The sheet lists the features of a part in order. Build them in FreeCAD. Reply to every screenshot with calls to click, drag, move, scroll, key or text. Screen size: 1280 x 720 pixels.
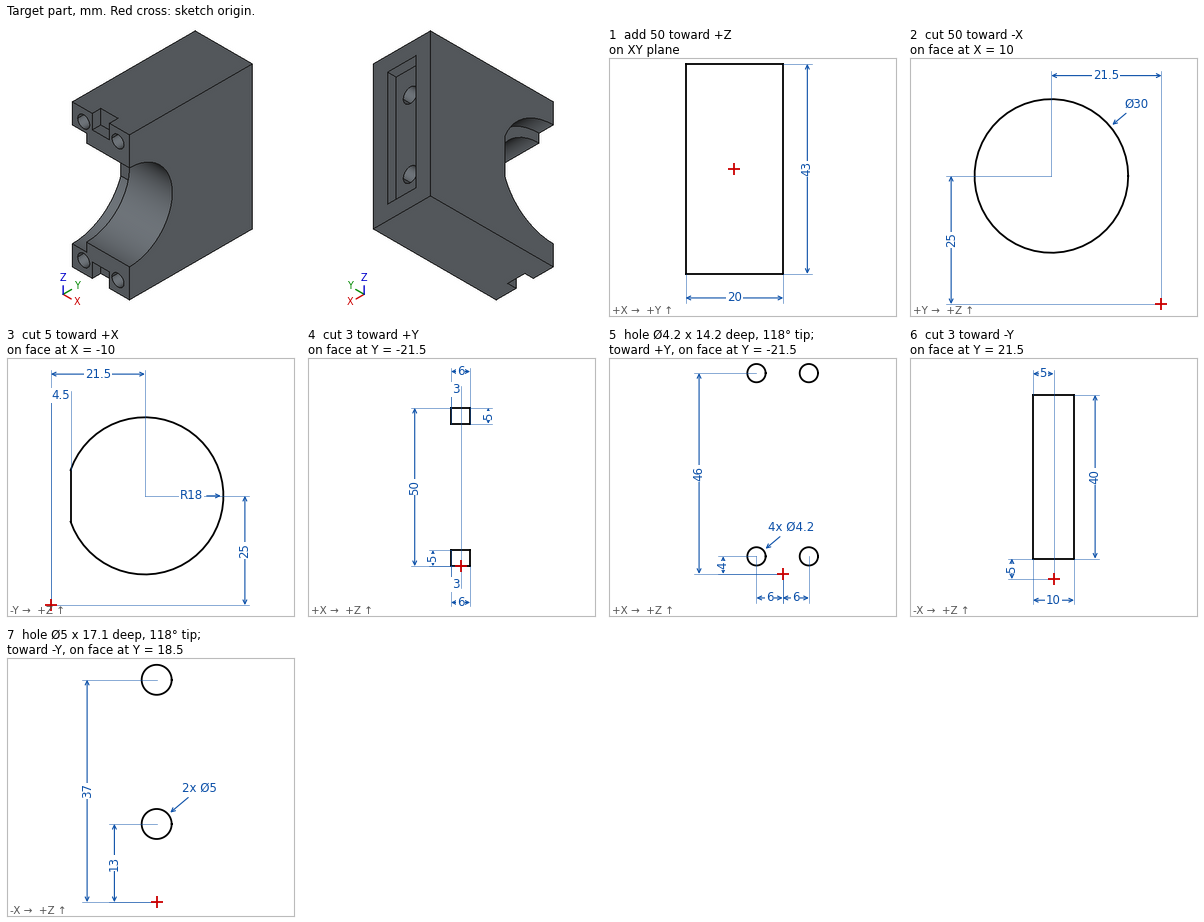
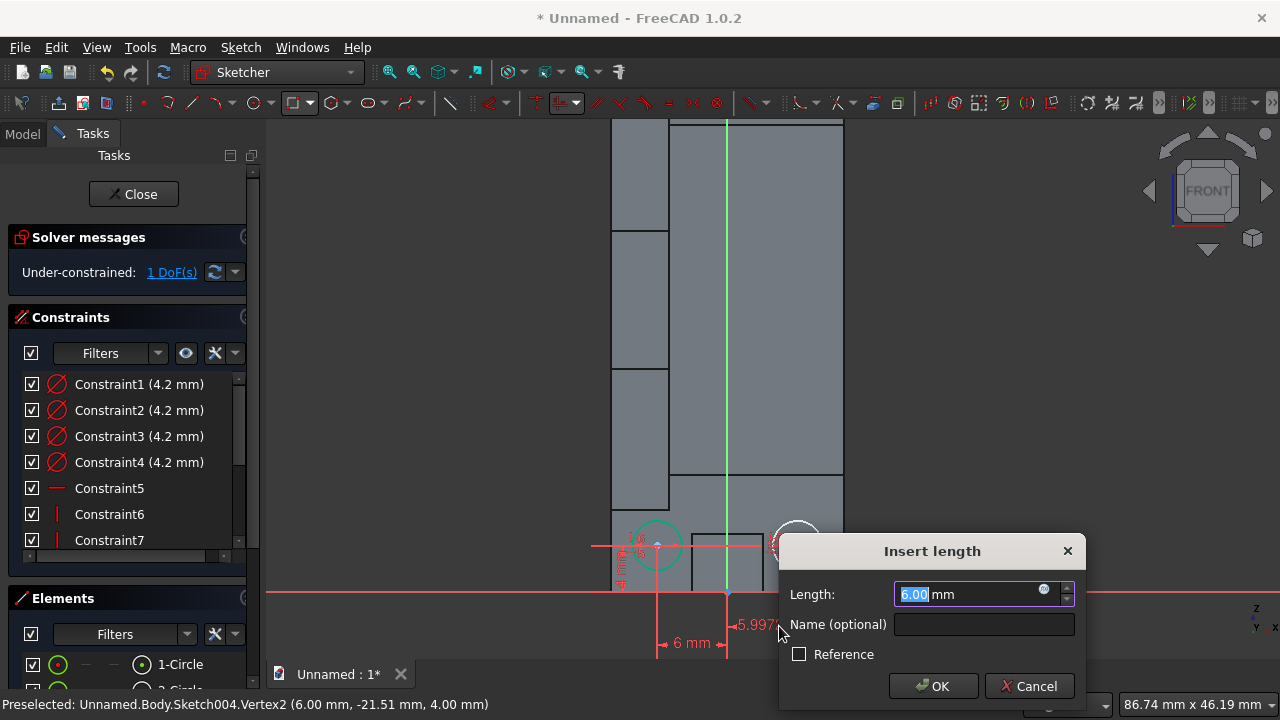
text(6)
key(Return)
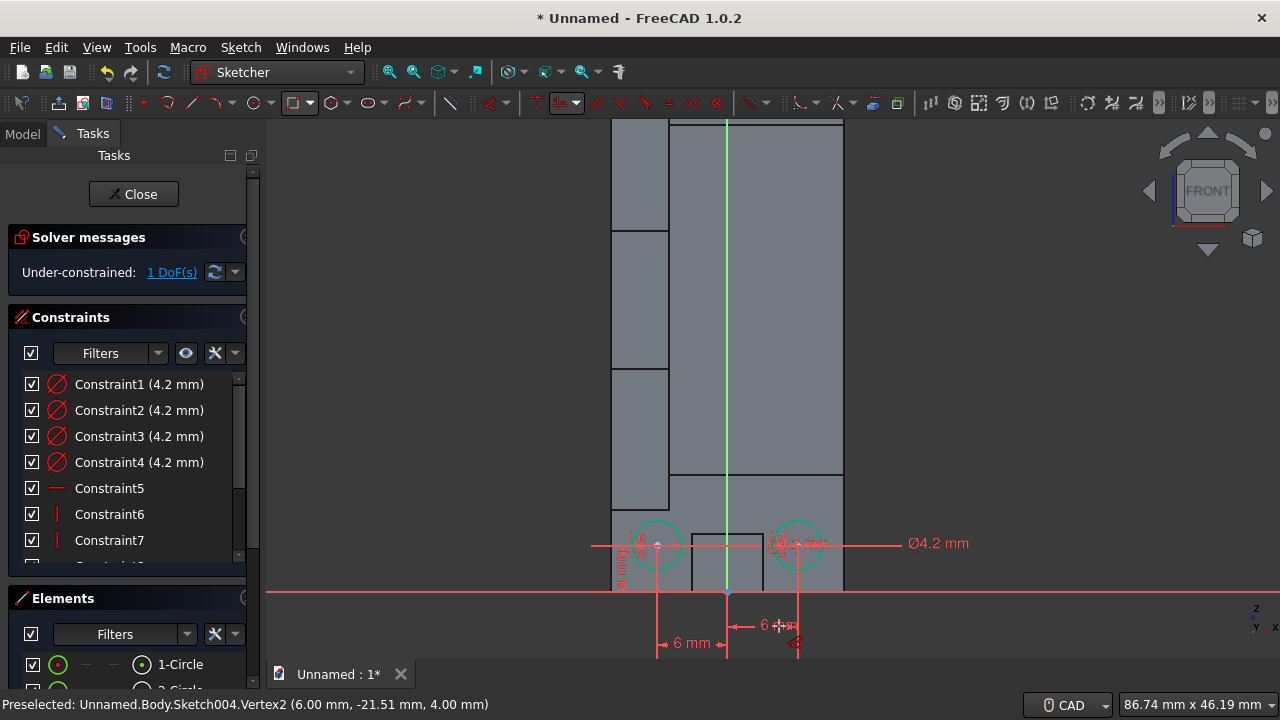
scroll(658, 547, down, 2)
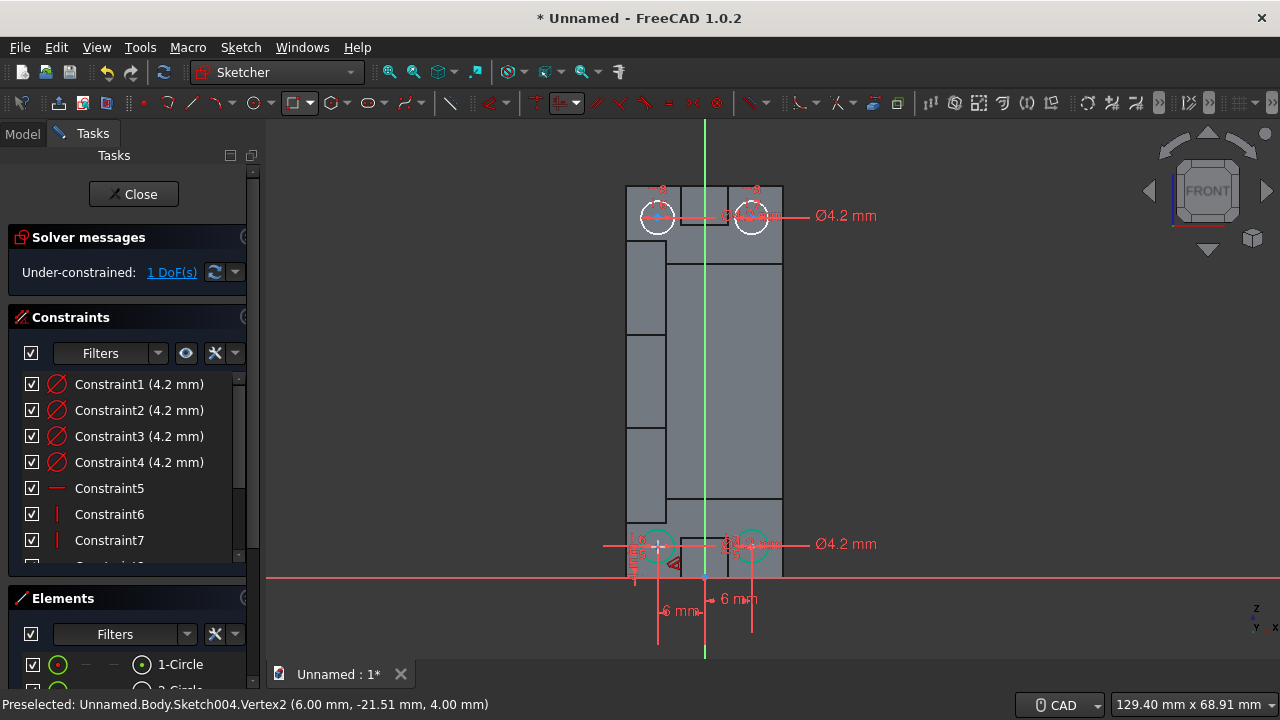
click(658, 218)
click(624, 398)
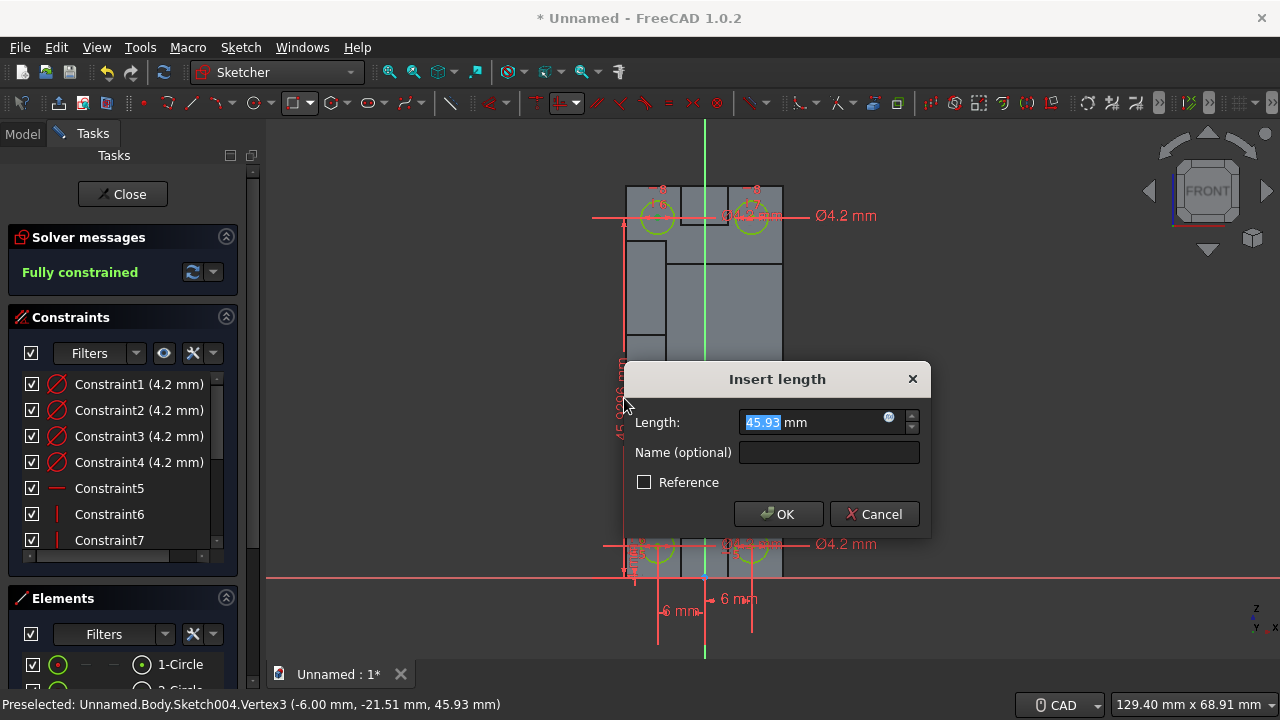
text(46)
key(Return)
key(Escape)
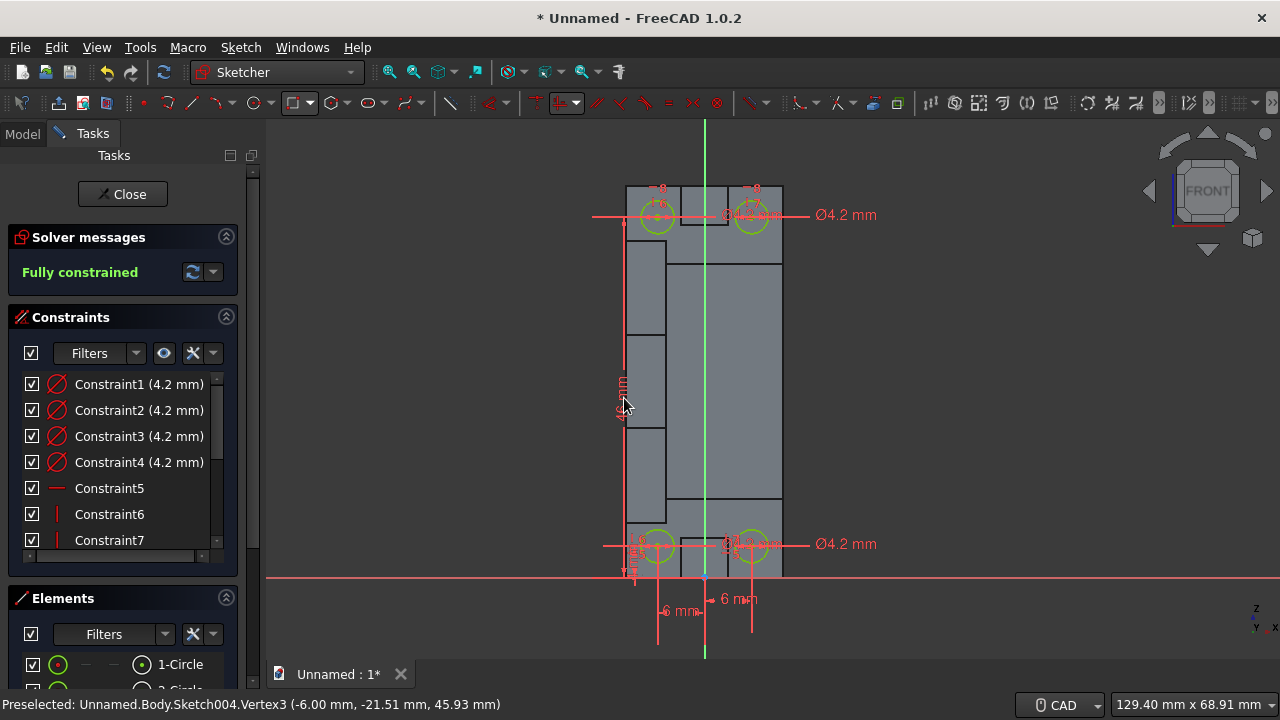
click(123, 194)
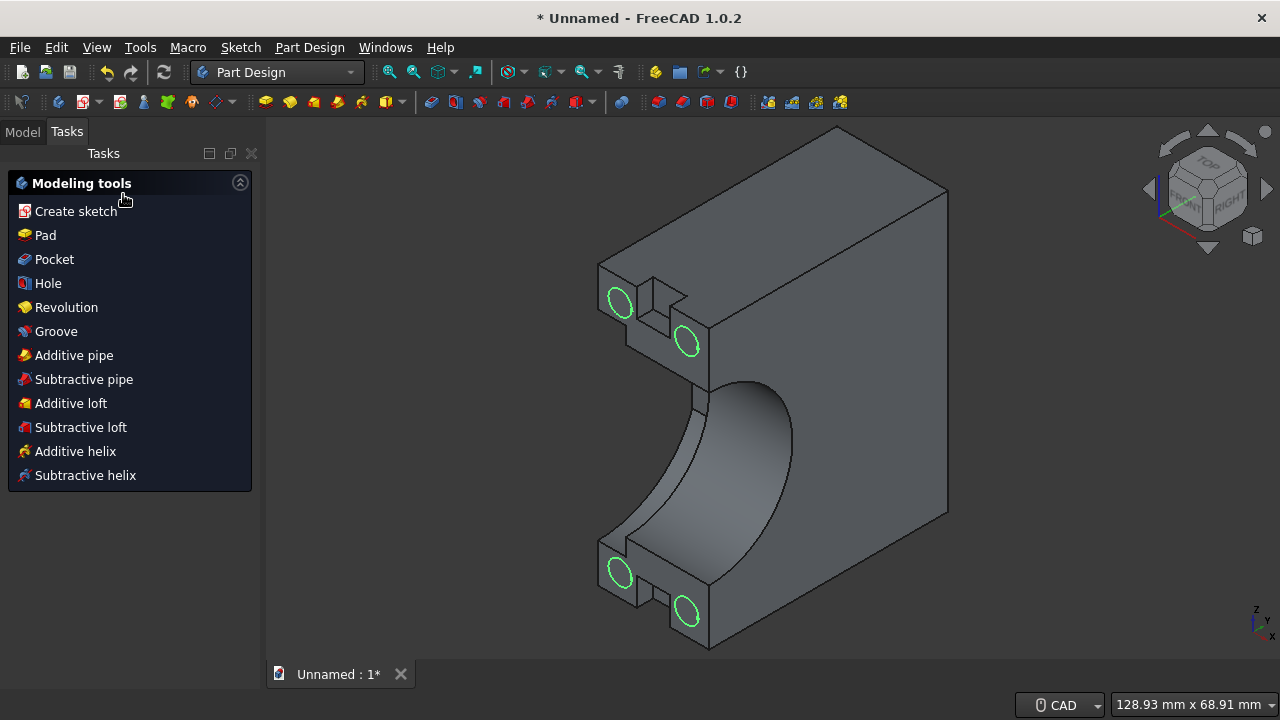
click(456, 102)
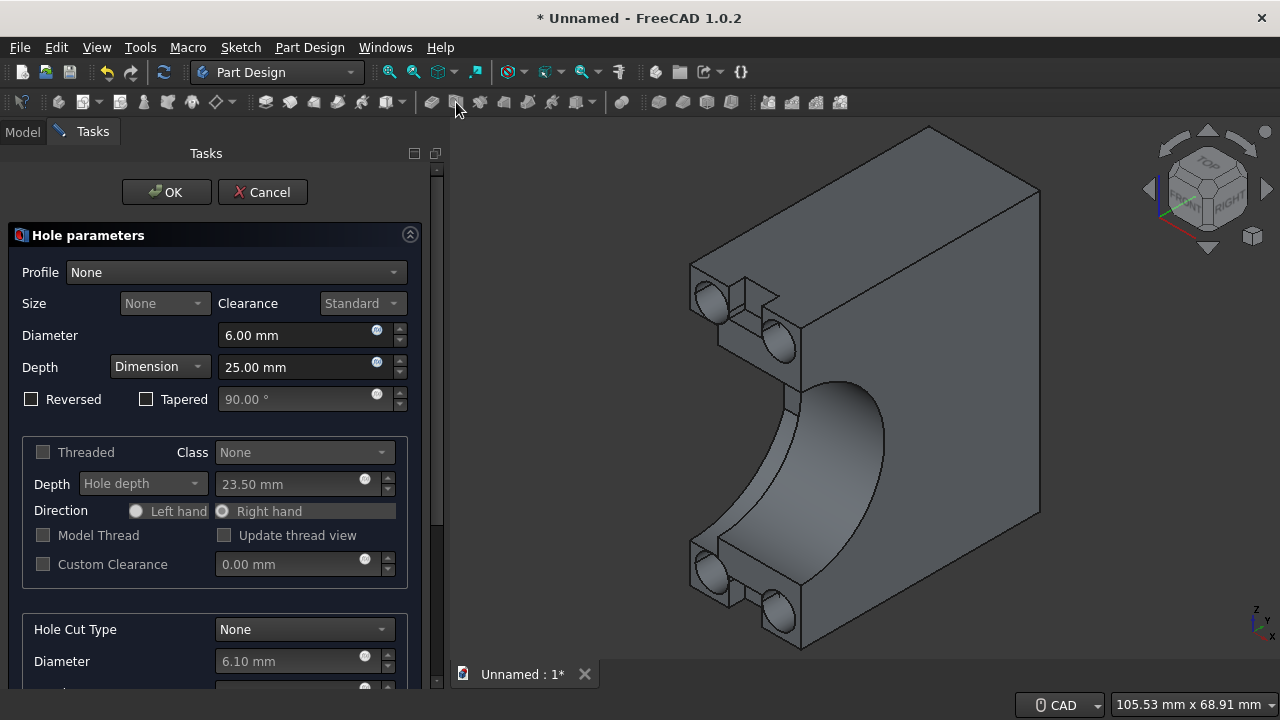
triple_click(305, 335)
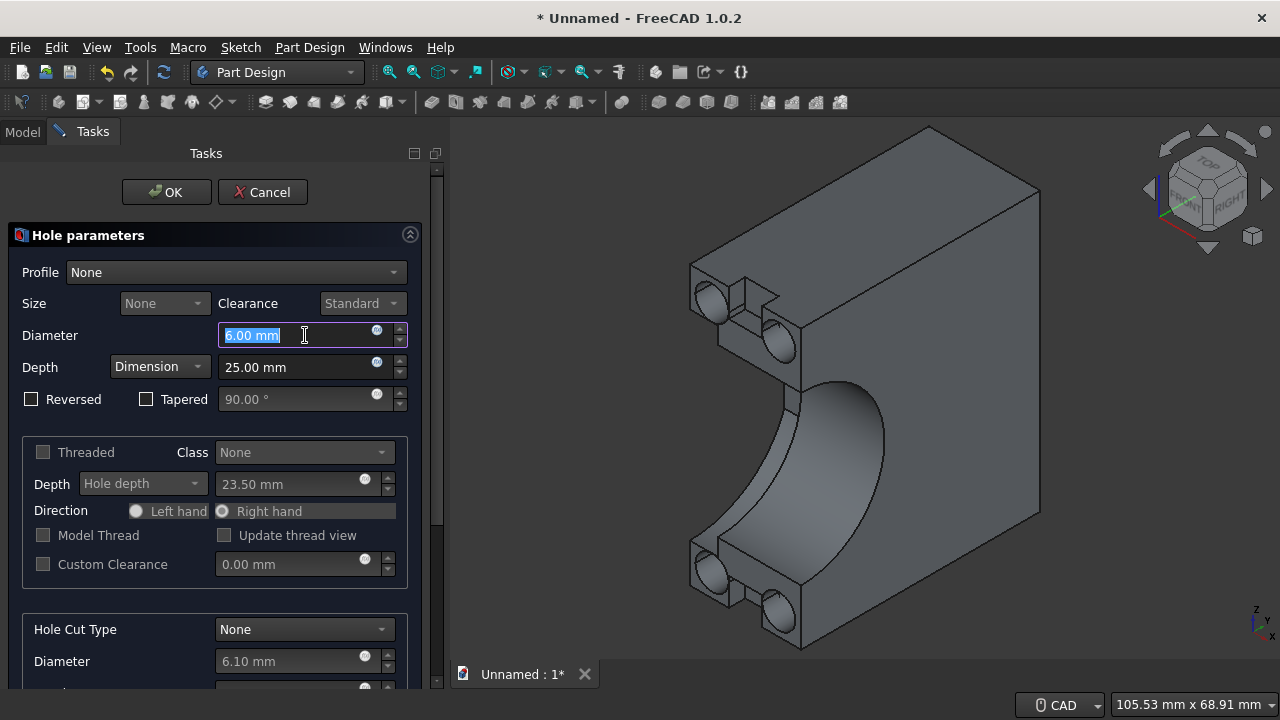
text(4.2)
key(Tab)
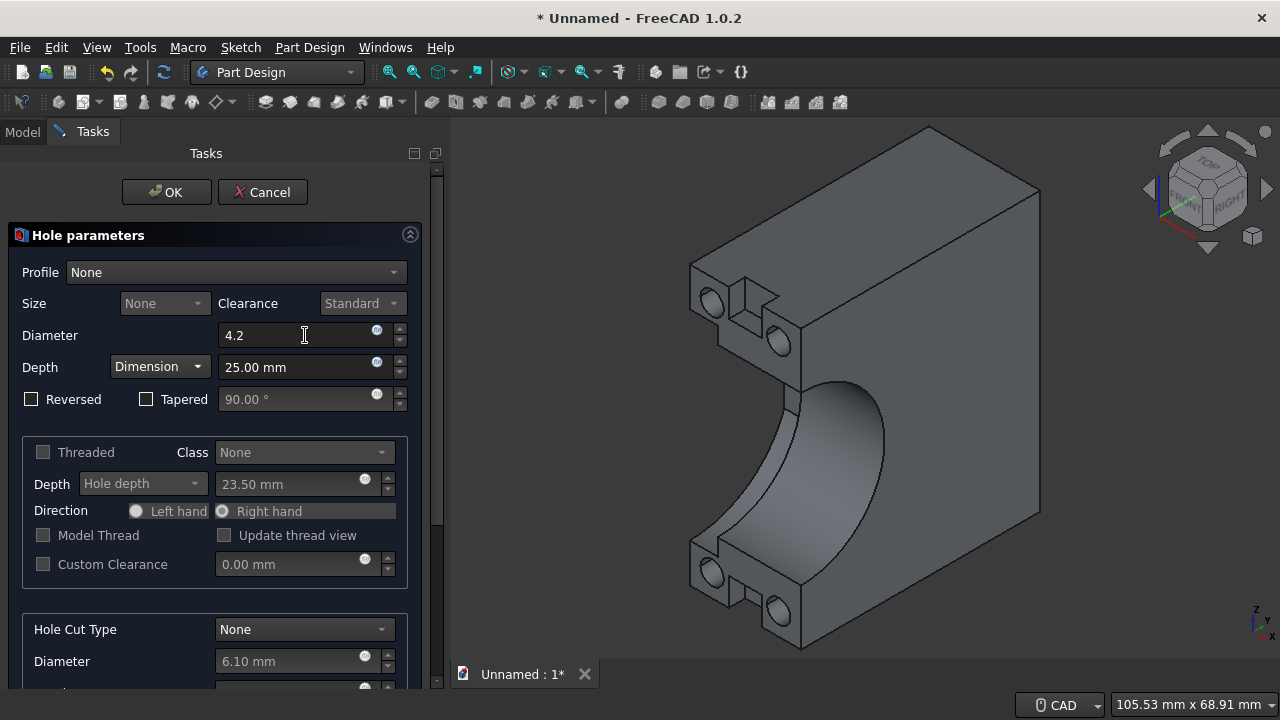
triple_click(305, 367)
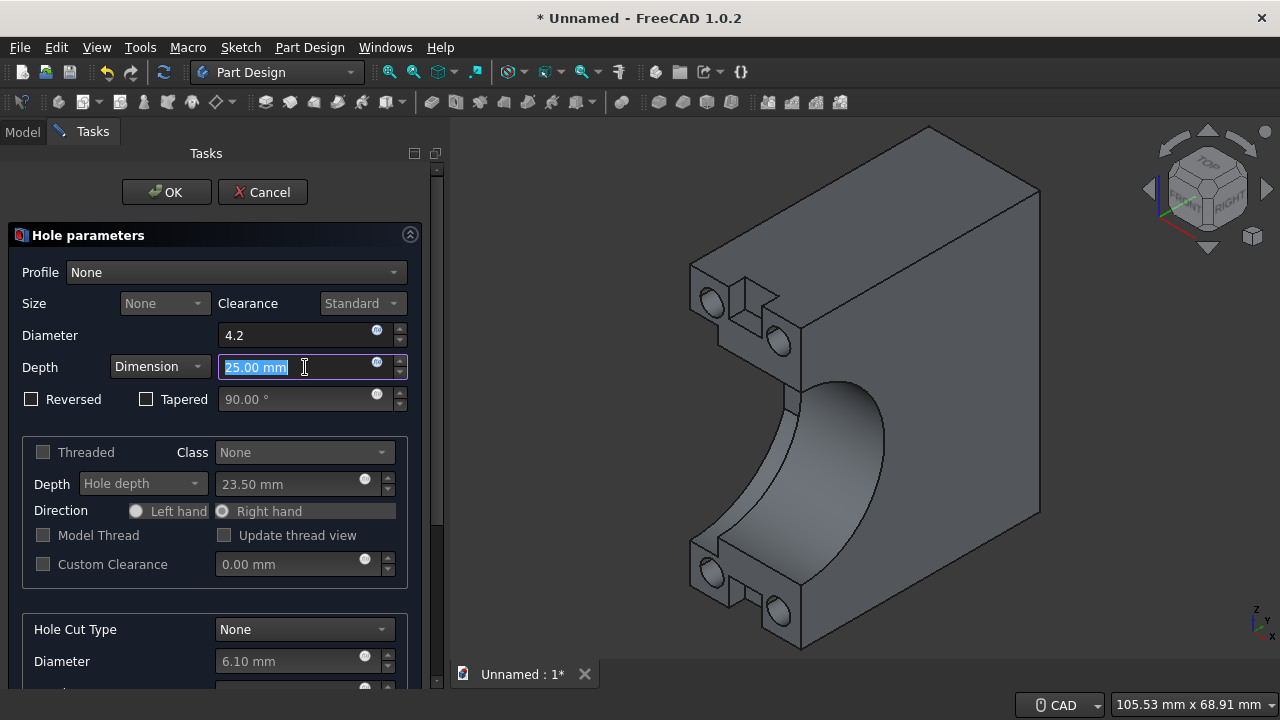
text(14.2)
key(Tab)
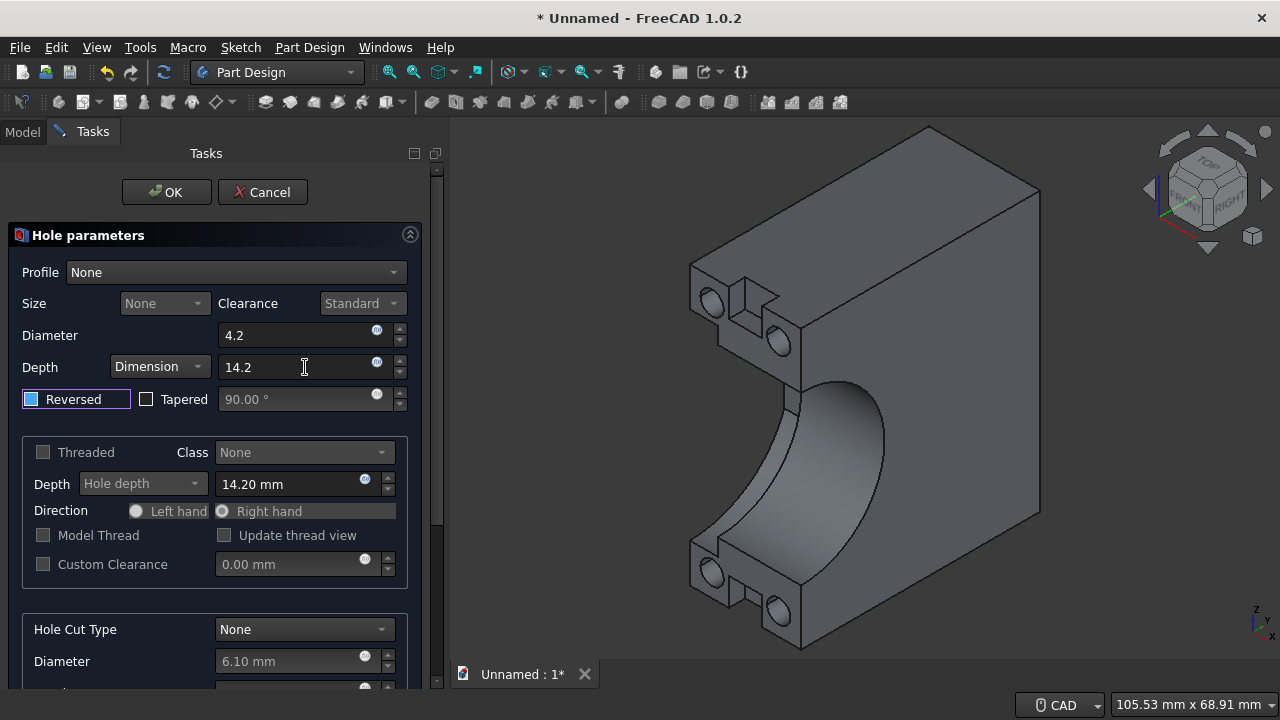
click(167, 192)